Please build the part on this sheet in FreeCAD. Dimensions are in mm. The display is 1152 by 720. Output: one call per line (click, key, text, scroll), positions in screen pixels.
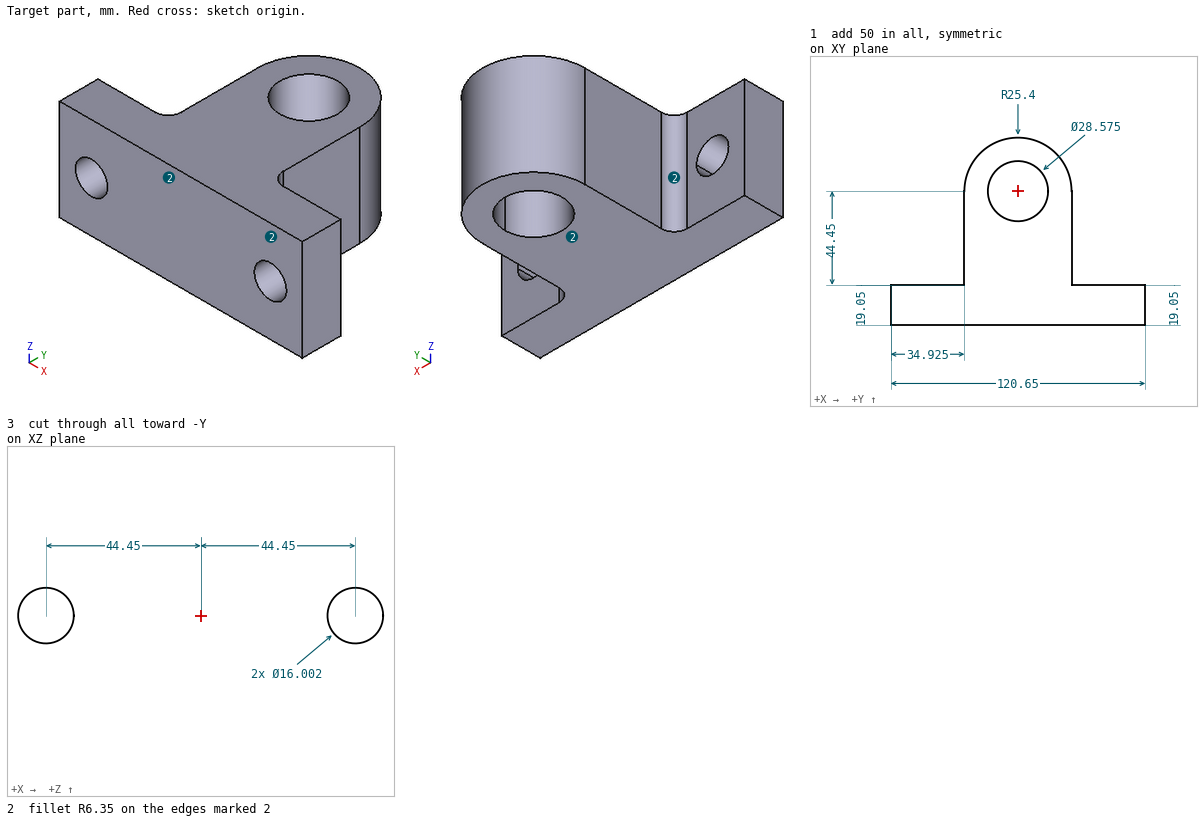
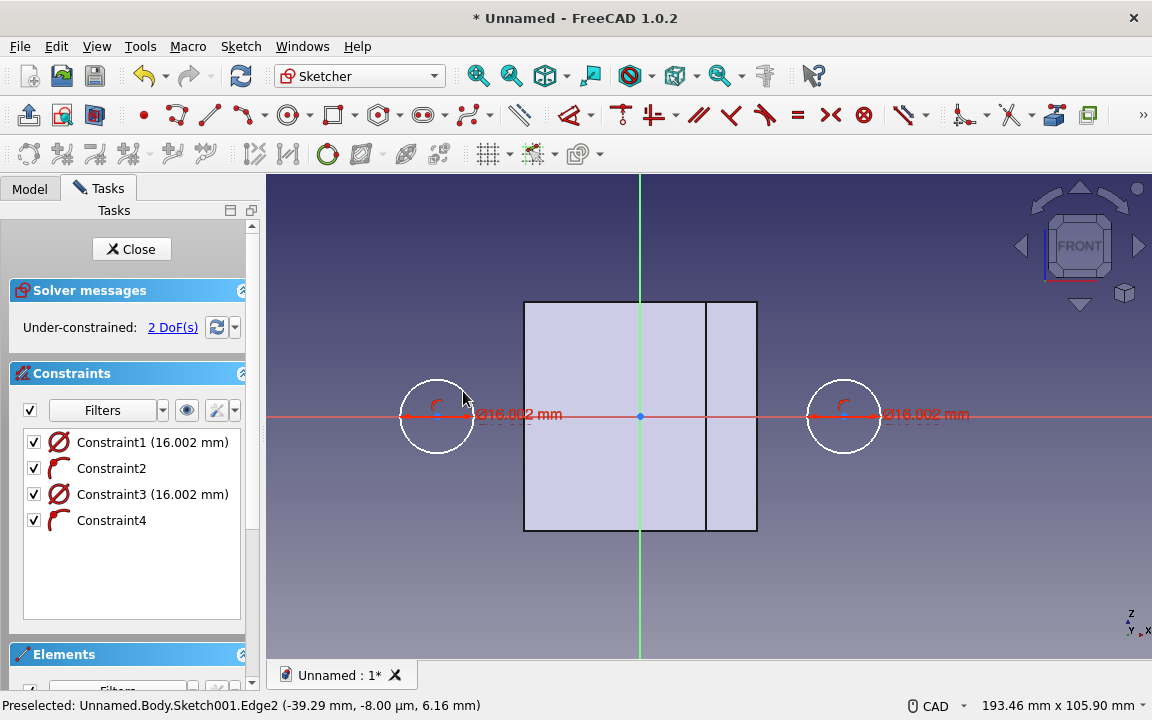
click(568, 116)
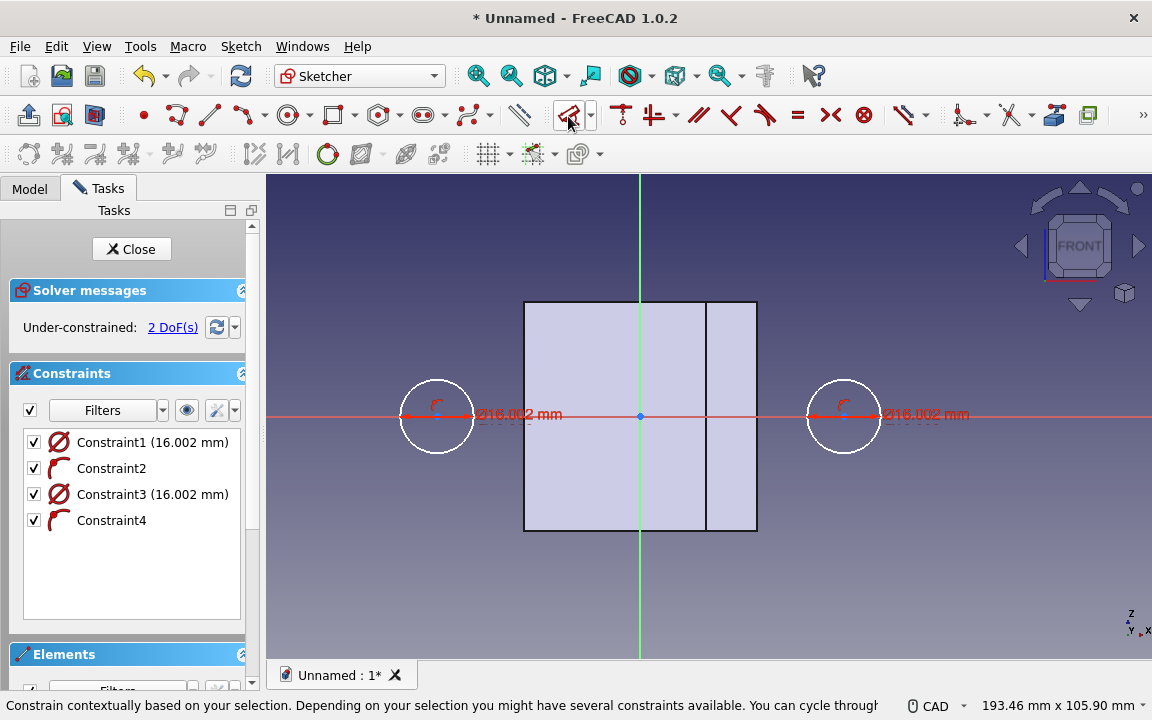
click(844, 416)
click(742, 450)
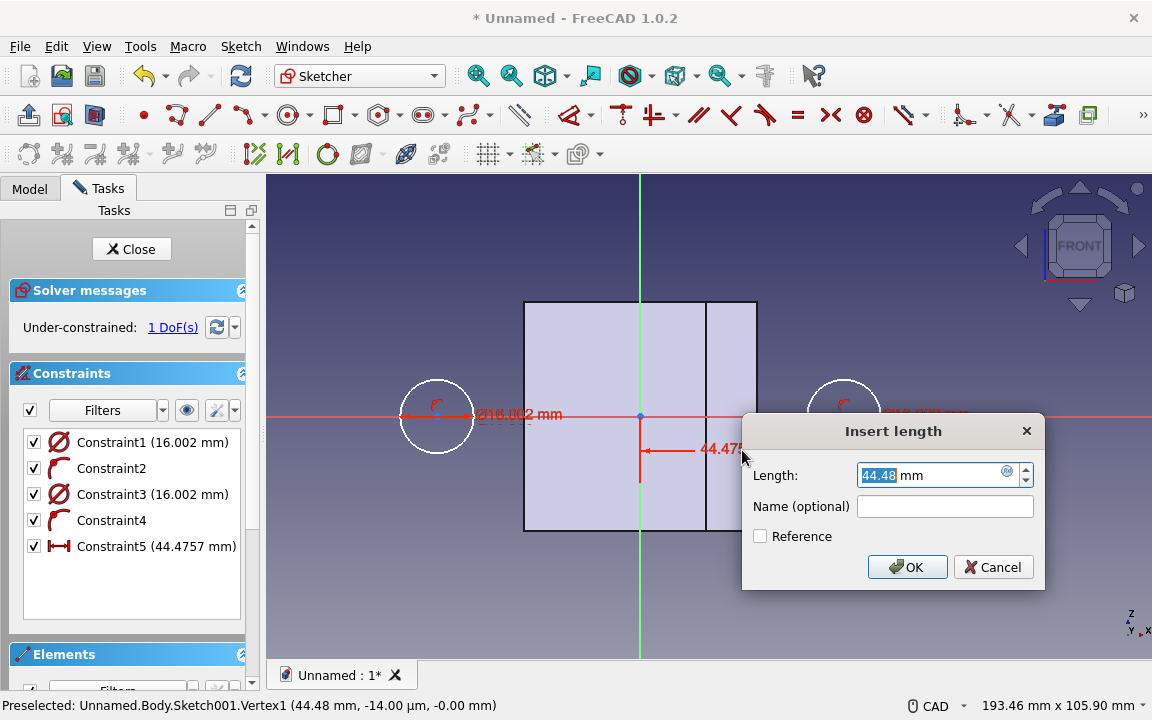
text(44.45)
key(Return)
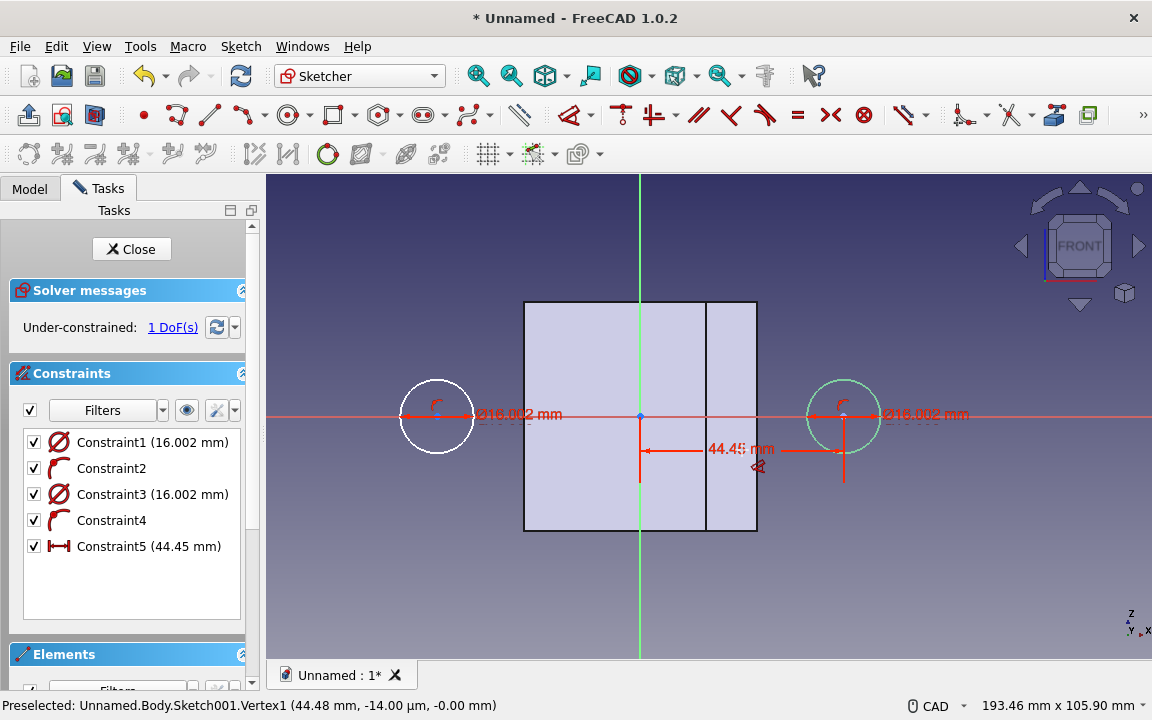
click(437, 416)
click(539, 450)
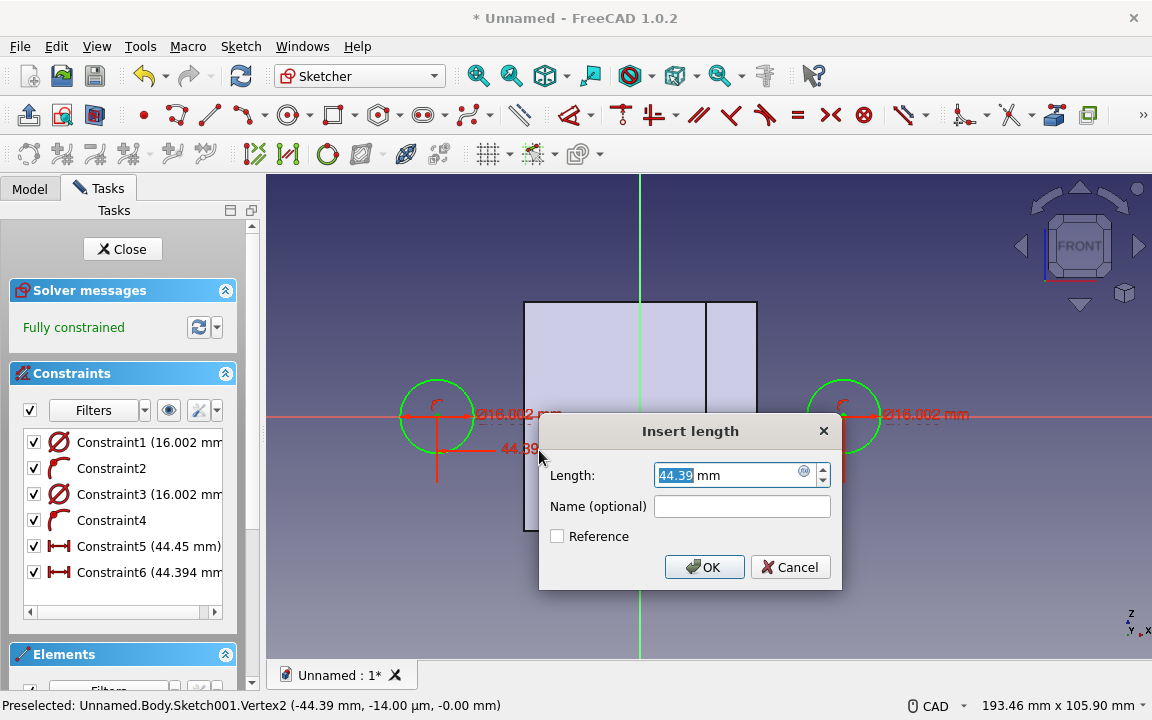
text(44.45)
key(Return)
key(Escape)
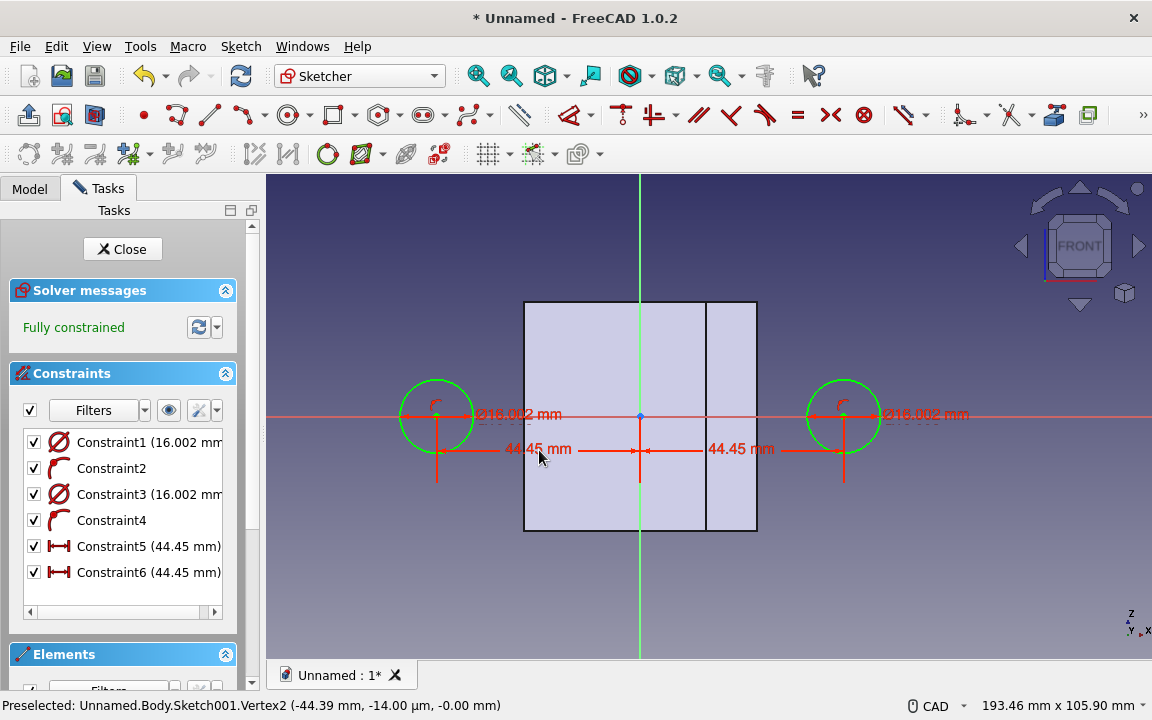
click(123, 249)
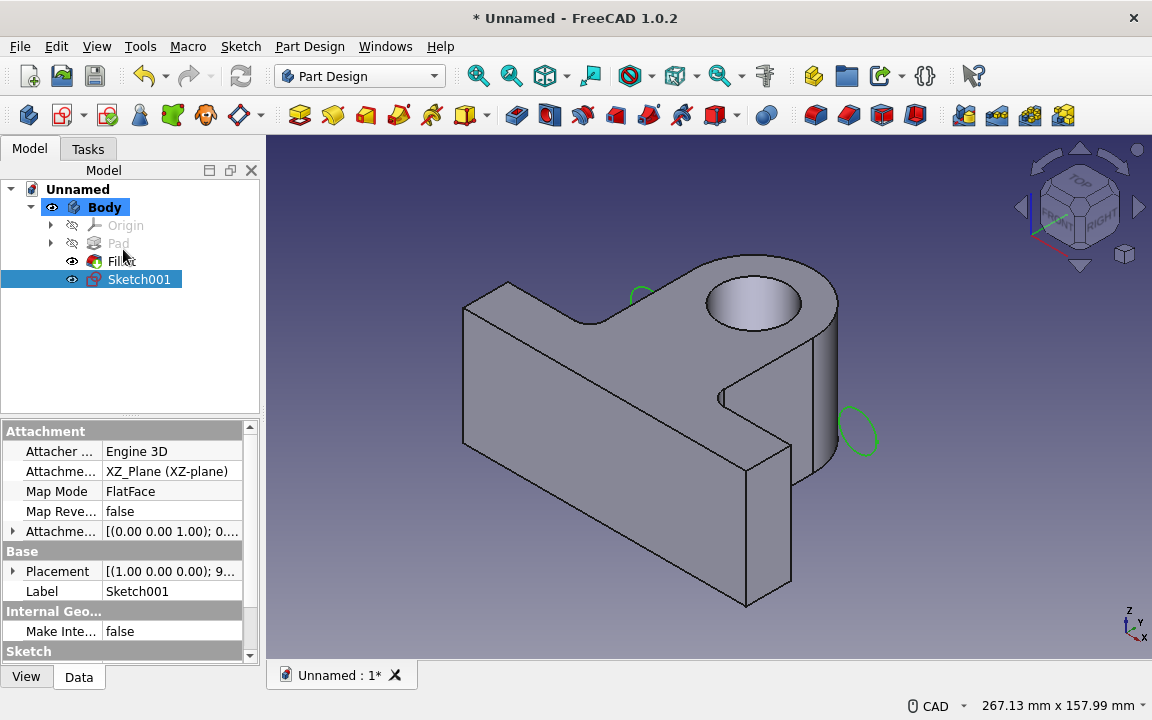
click(517, 116)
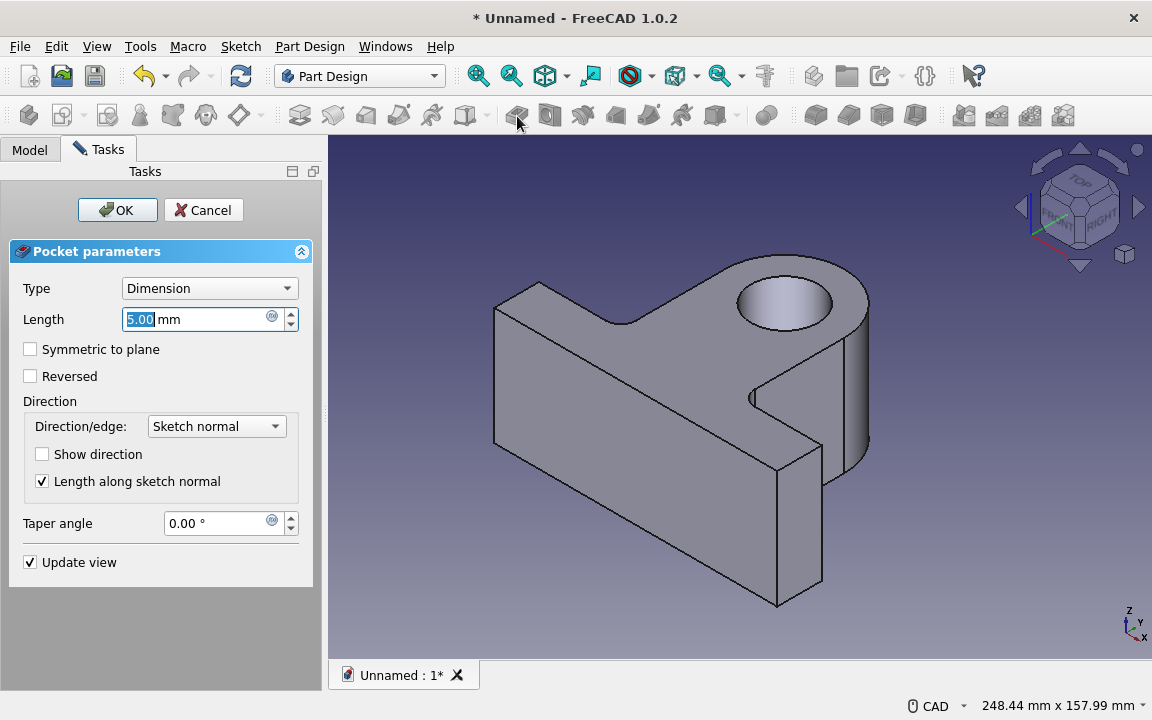
click(210, 288)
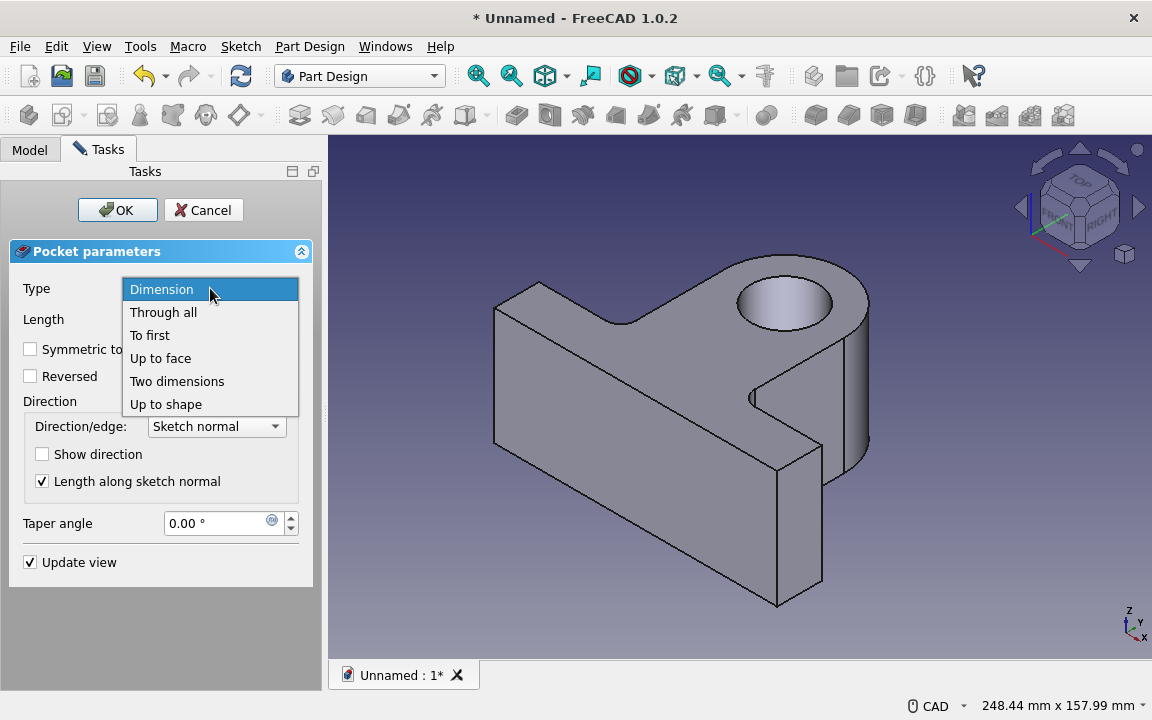
click(208, 312)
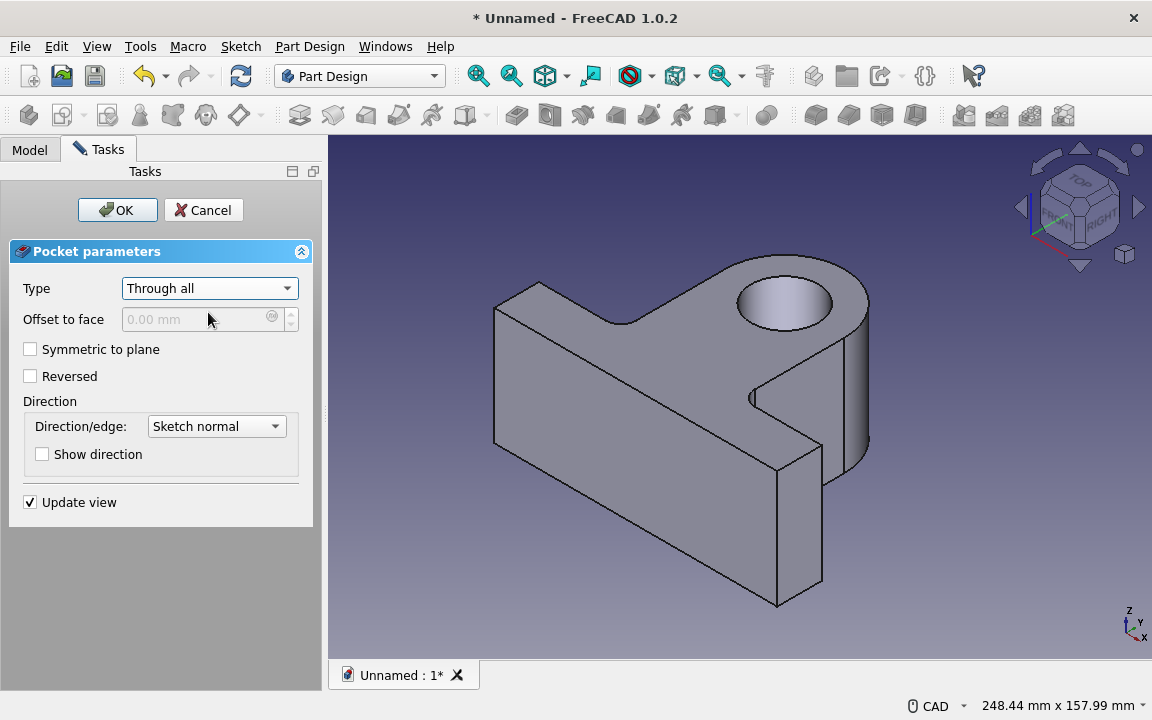
click(31, 376)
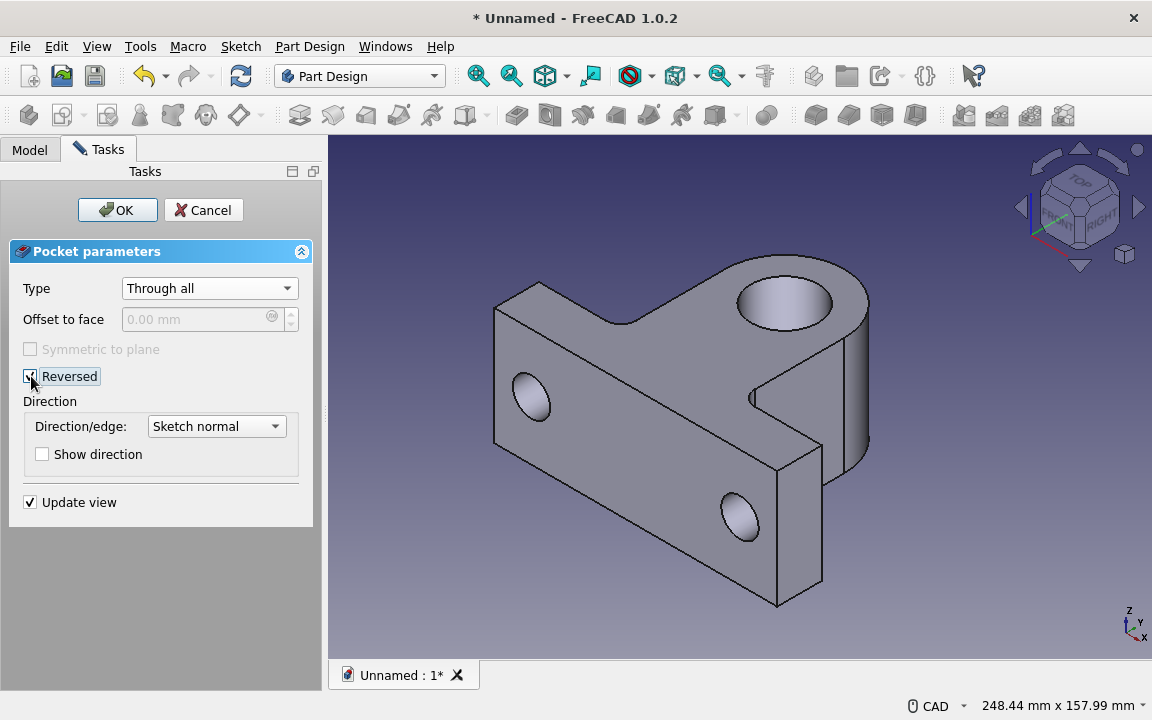
click(118, 210)